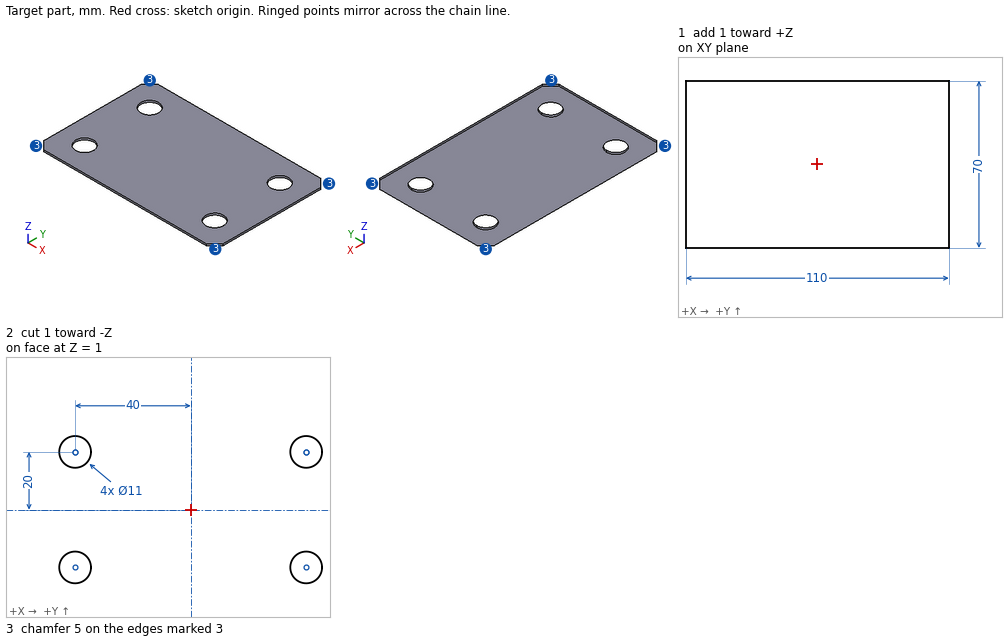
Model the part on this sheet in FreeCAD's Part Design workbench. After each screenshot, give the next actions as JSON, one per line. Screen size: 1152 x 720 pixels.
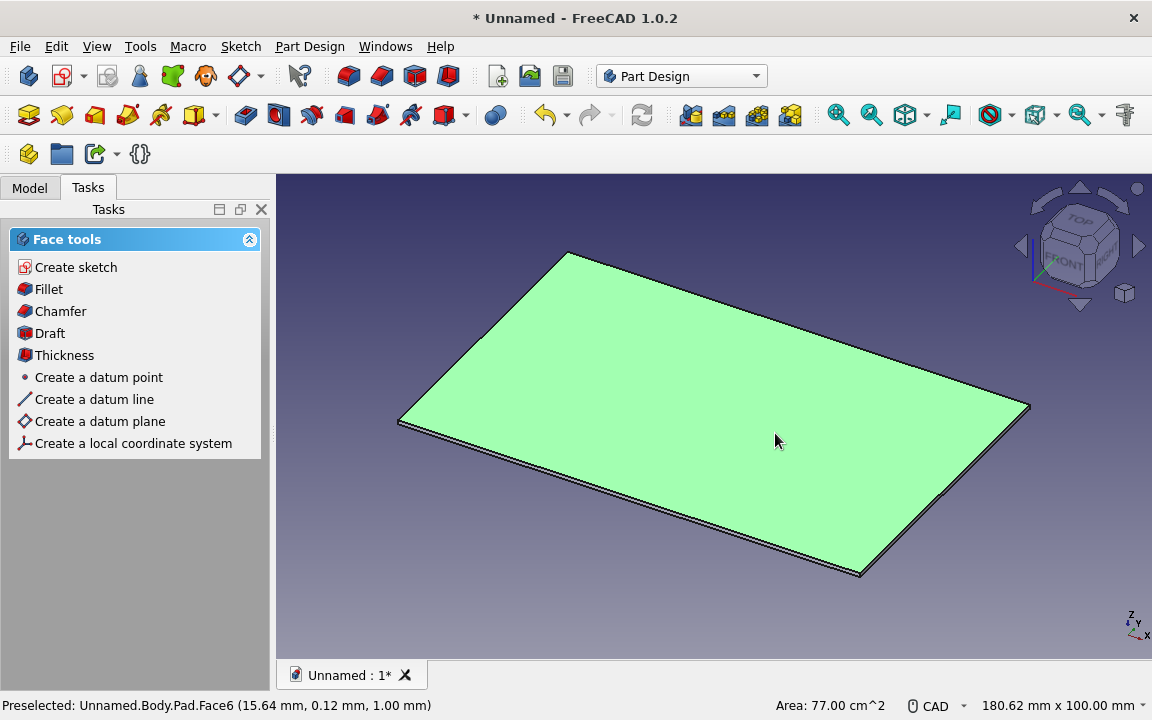
{"action": "left_click", "coordinate": [62, 76]}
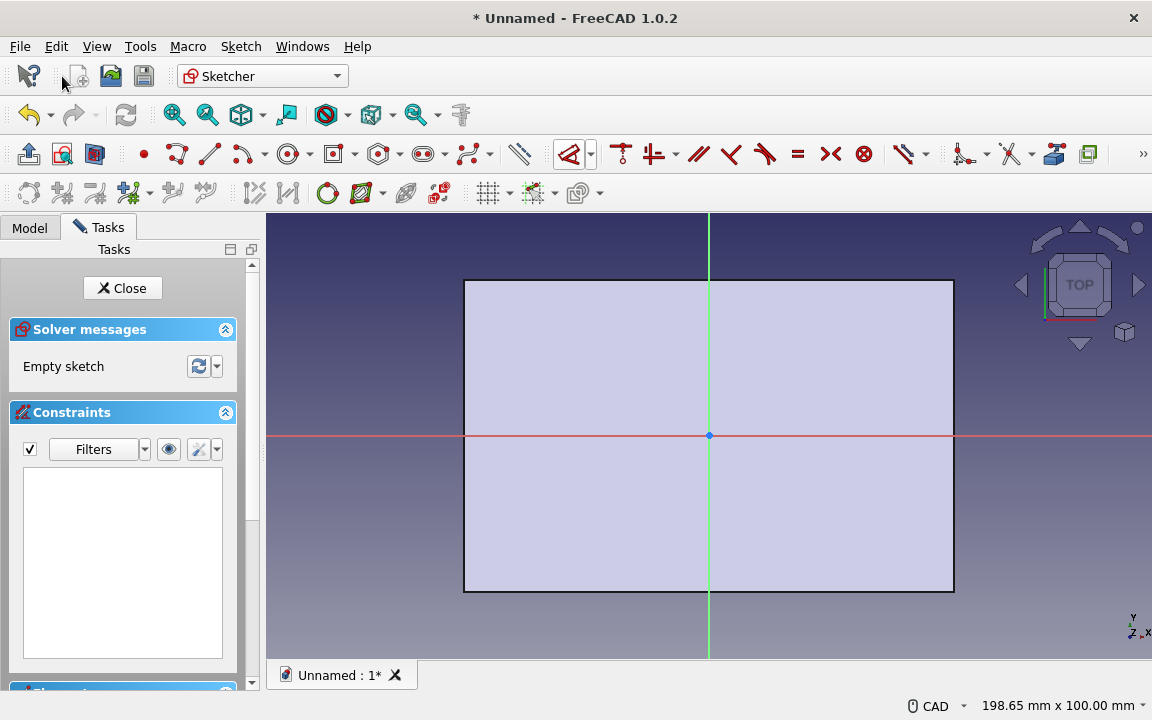
{"action": "left_click", "coordinate": [288, 154]}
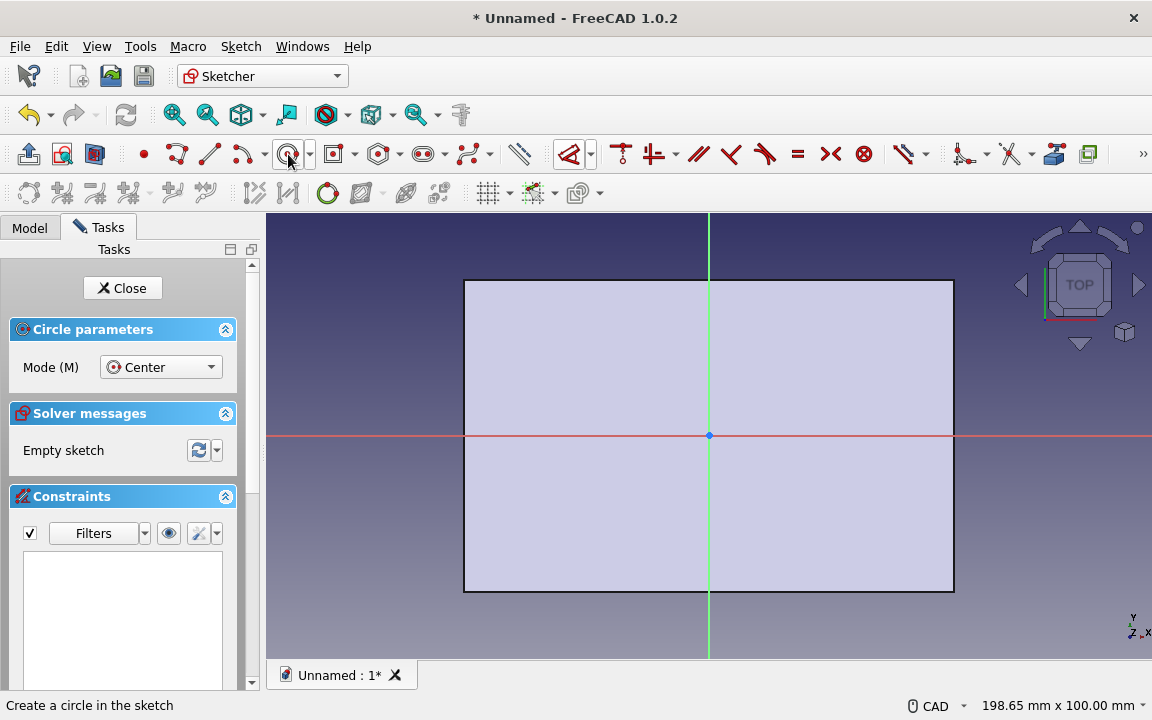
{"action": "left_click", "coordinate": [531, 347]}
{"action": "mouse_move", "coordinate": [548, 329]}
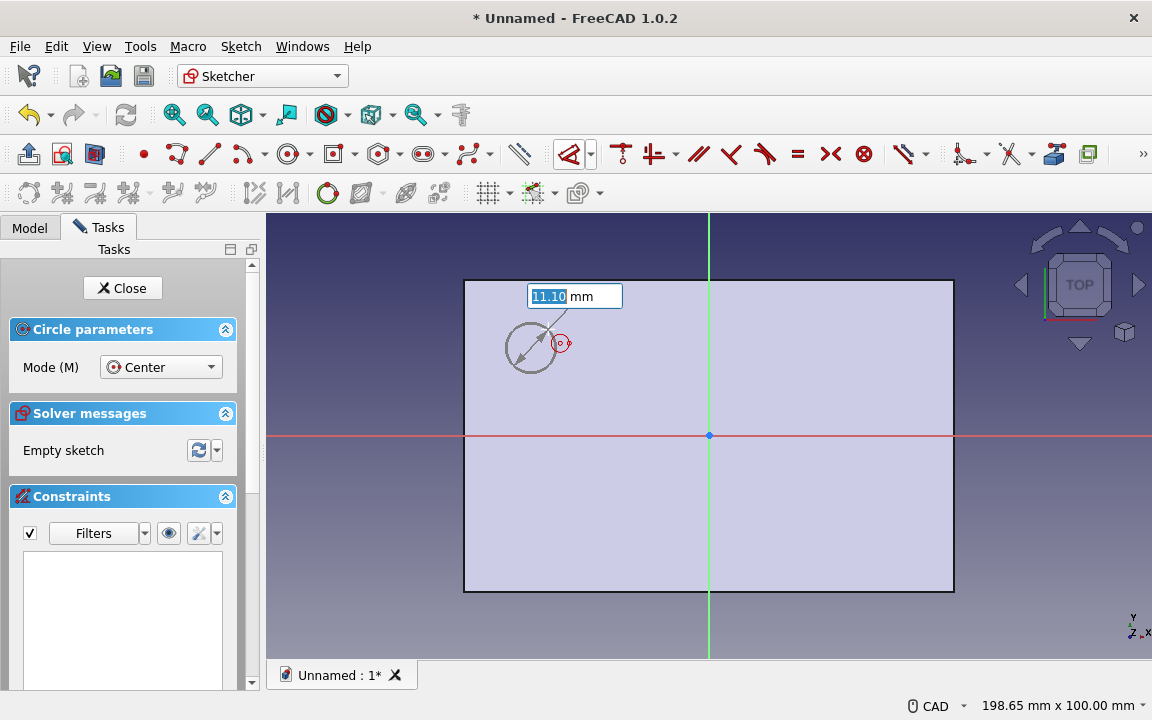
{"action": "type", "text": "11"}
{"action": "key", "text": "Return"}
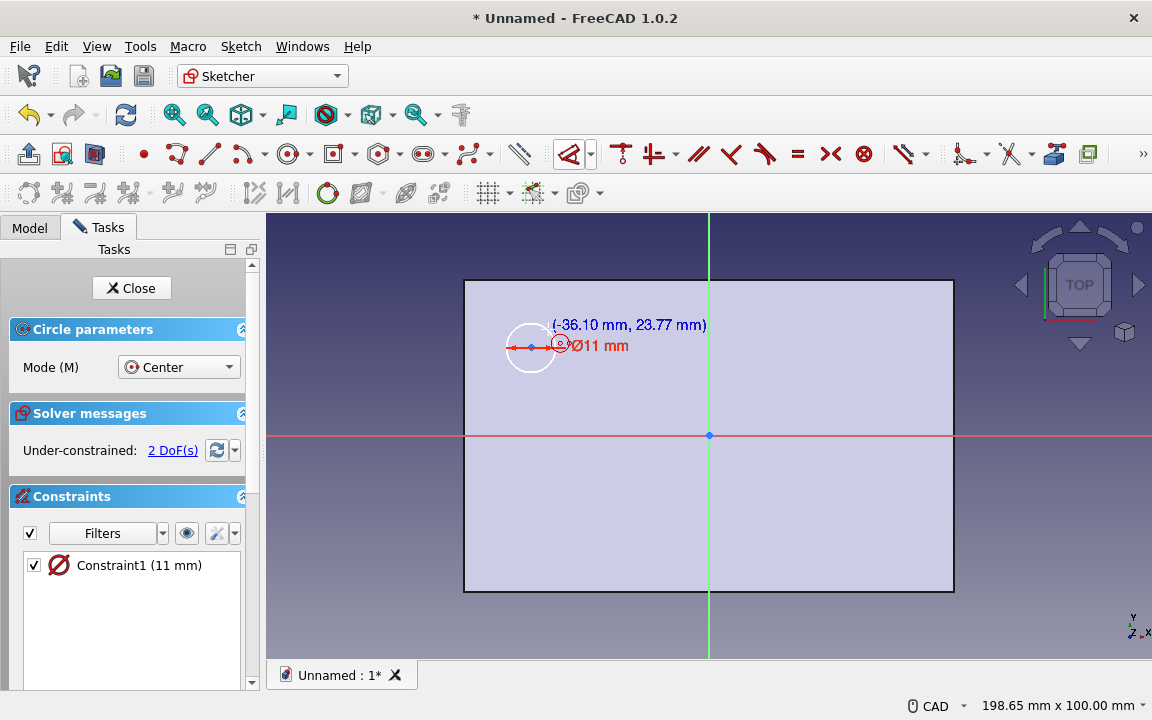
{"action": "left_click", "coordinate": [887, 347]}
{"action": "mouse_move", "coordinate": [905, 329]}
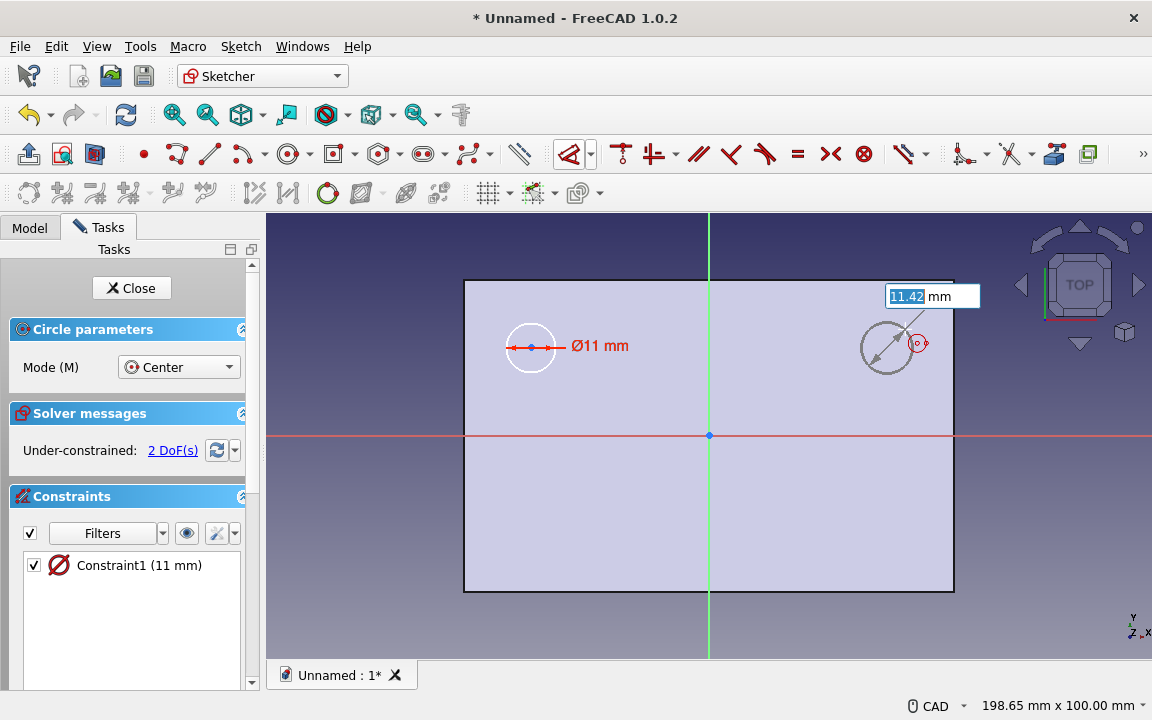
{"action": "type", "text": "11"}
{"action": "key", "text": "Return"}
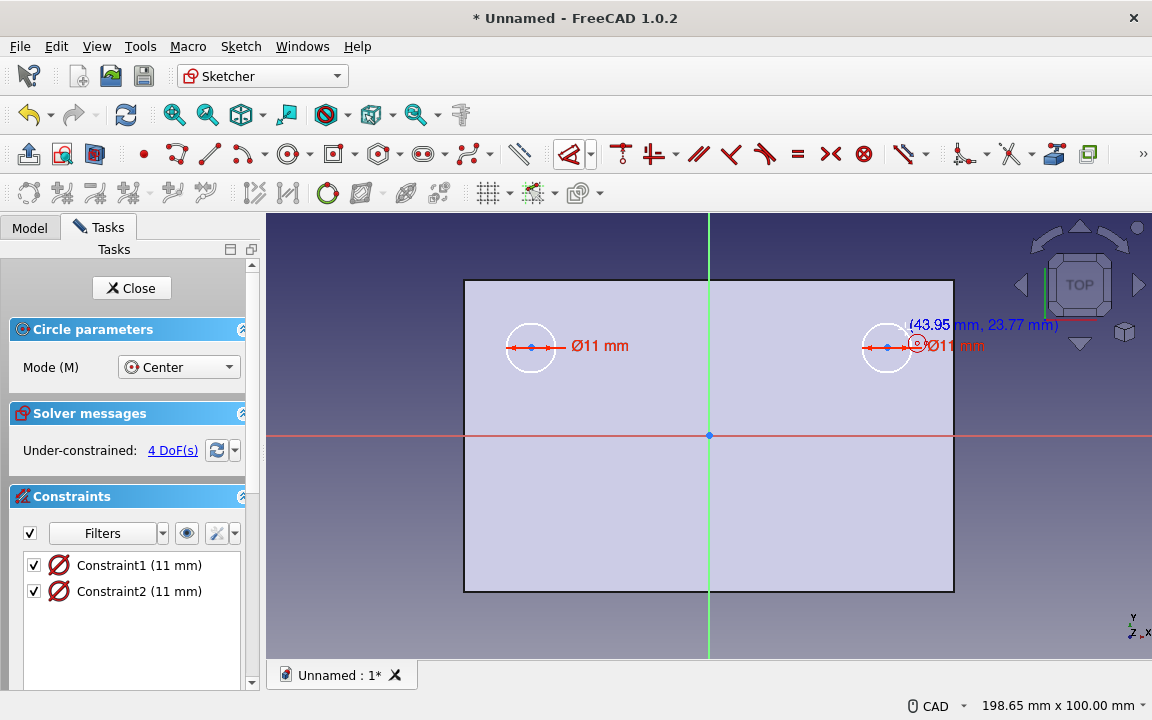
{"action": "left_click", "coordinate": [531, 525]}
{"action": "mouse_move", "coordinate": [548, 508]}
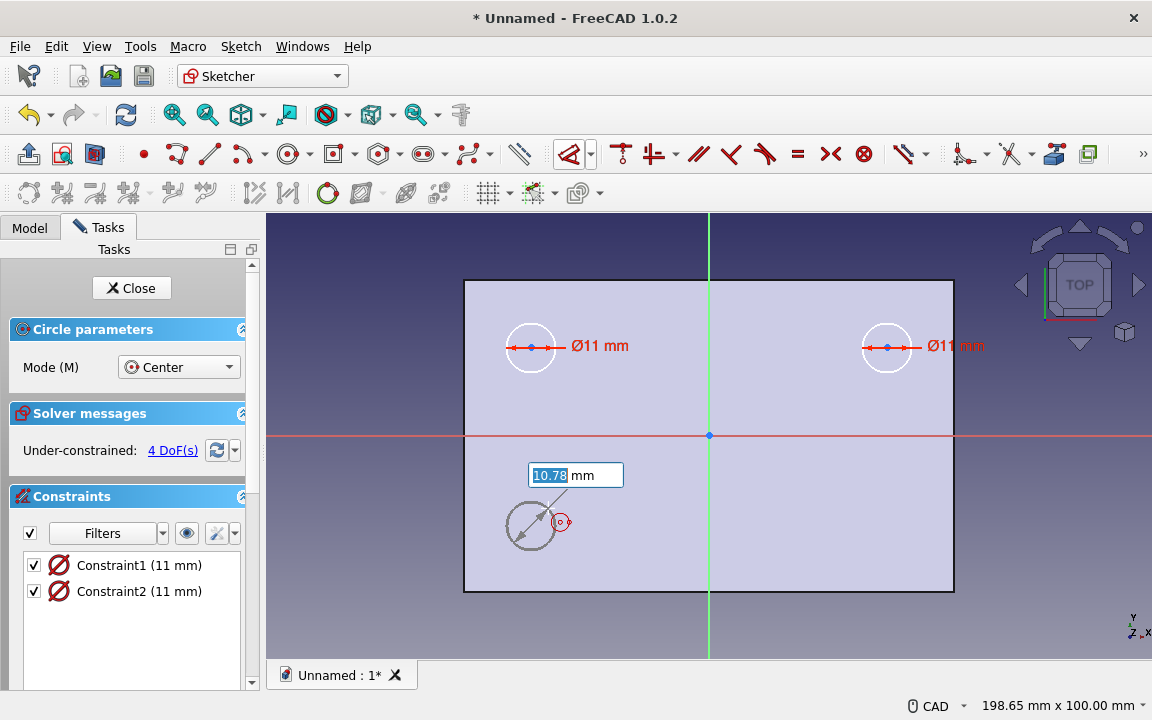
{"action": "type", "text": "11"}
{"action": "key", "text": "Return"}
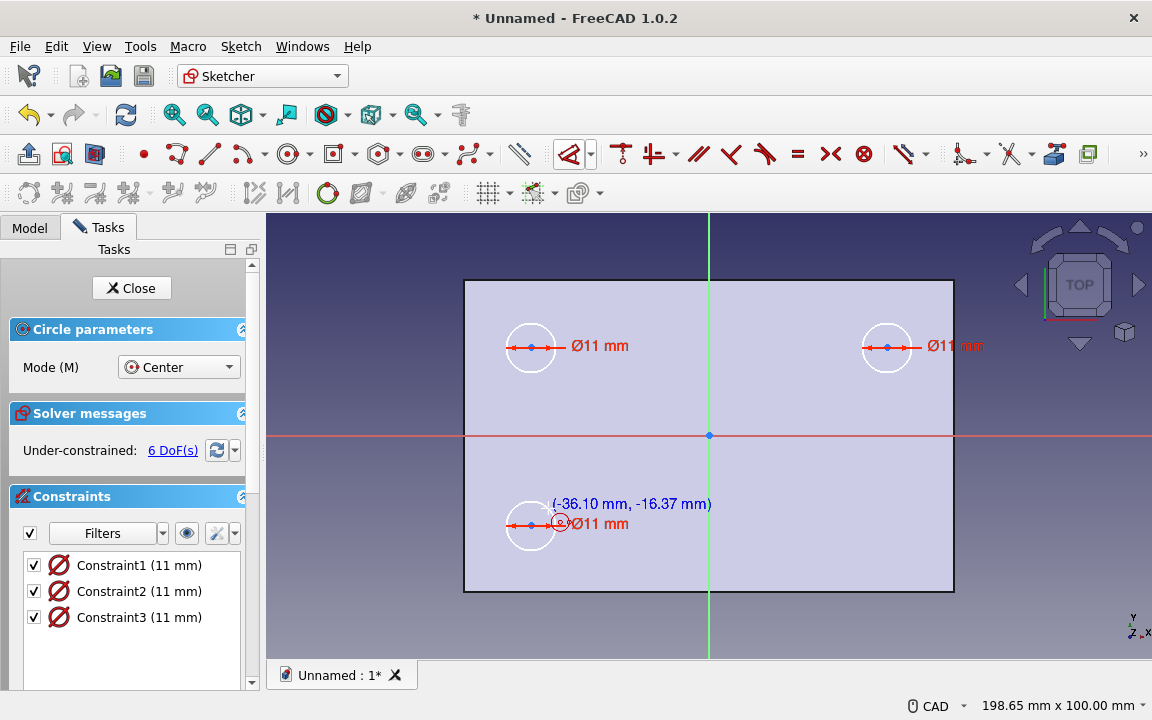
{"action": "left_click", "coordinate": [887, 525]}
{"action": "mouse_move", "coordinate": [905, 508]}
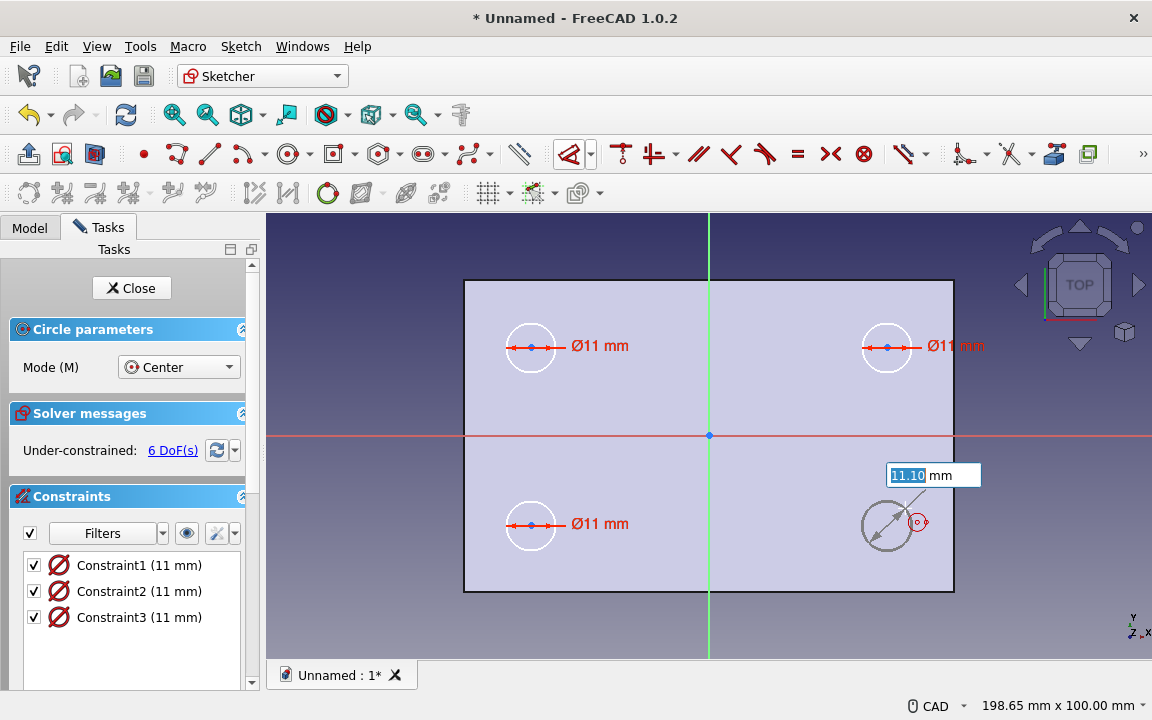
{"action": "type", "text": "11"}
{"action": "key", "text": "Return"}
{"action": "key", "text": "Escape"}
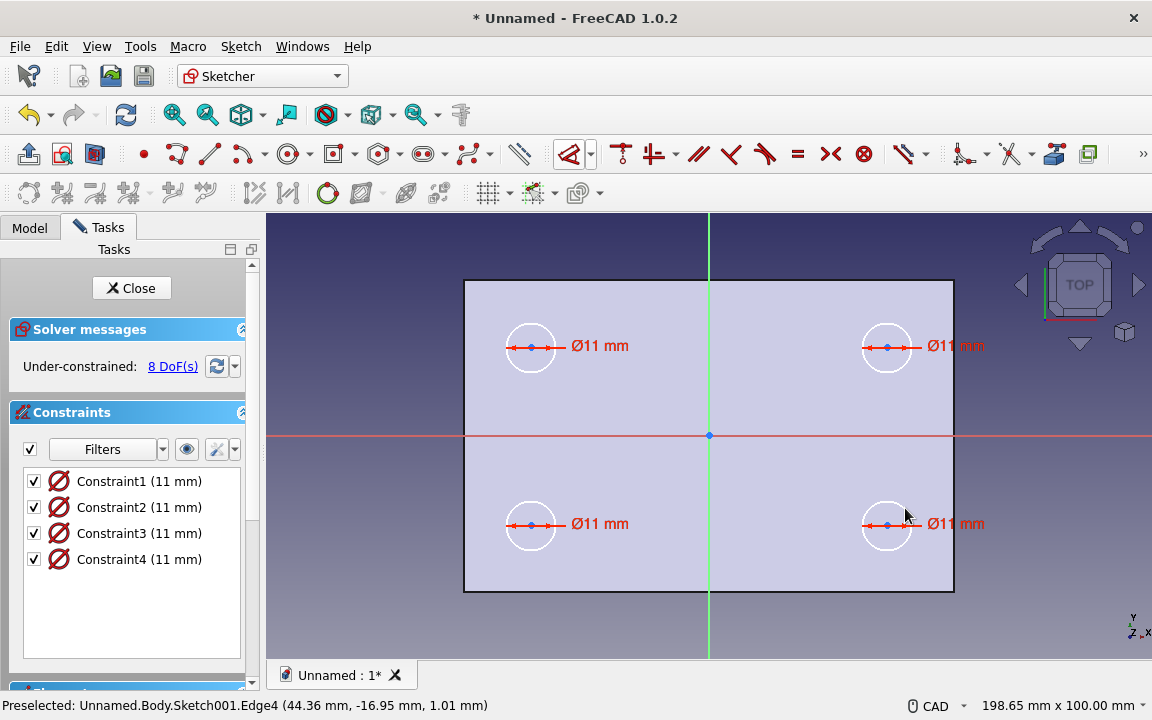
{"action": "left_click", "coordinate": [531, 348]}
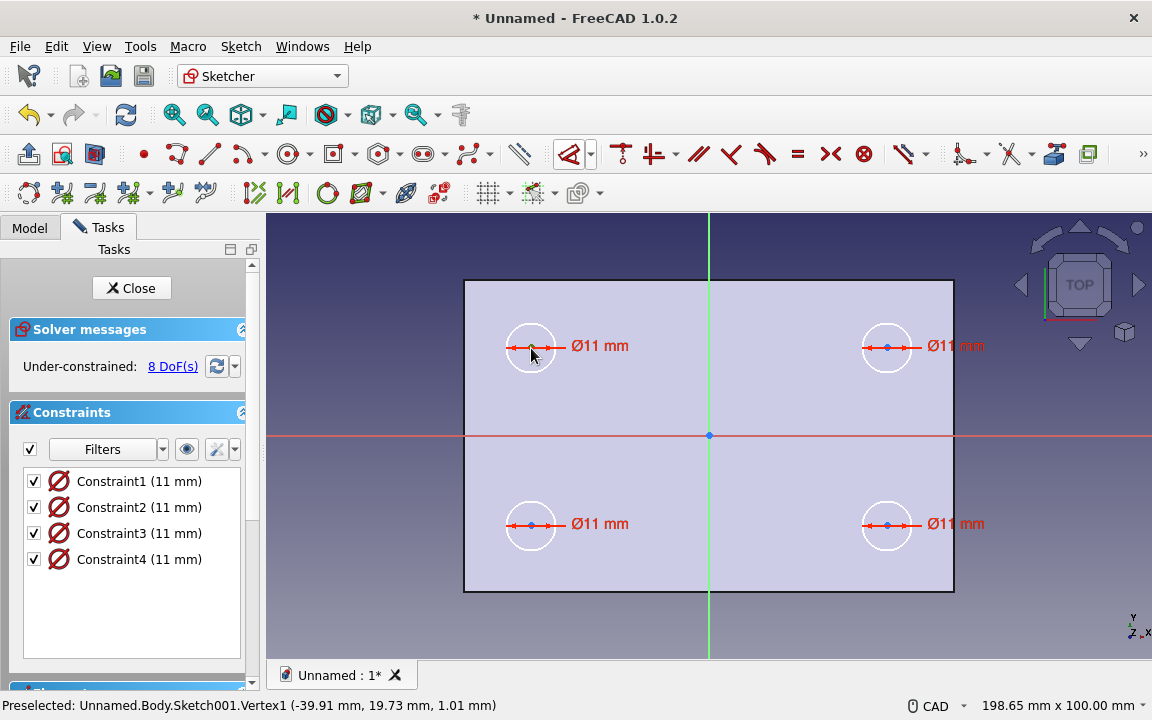
{"action": "left_click", "coordinate": [887, 348]}